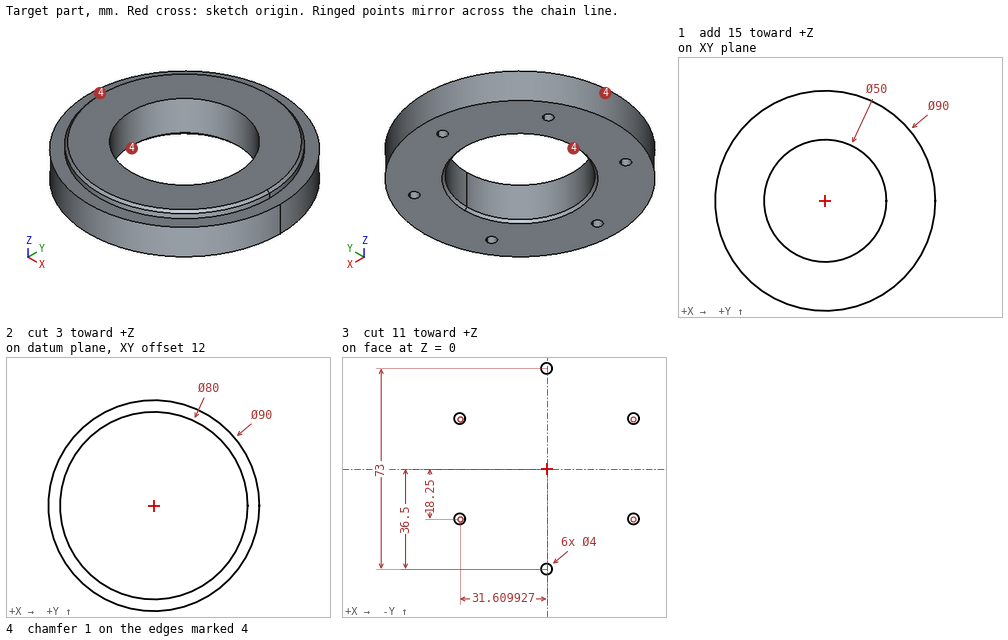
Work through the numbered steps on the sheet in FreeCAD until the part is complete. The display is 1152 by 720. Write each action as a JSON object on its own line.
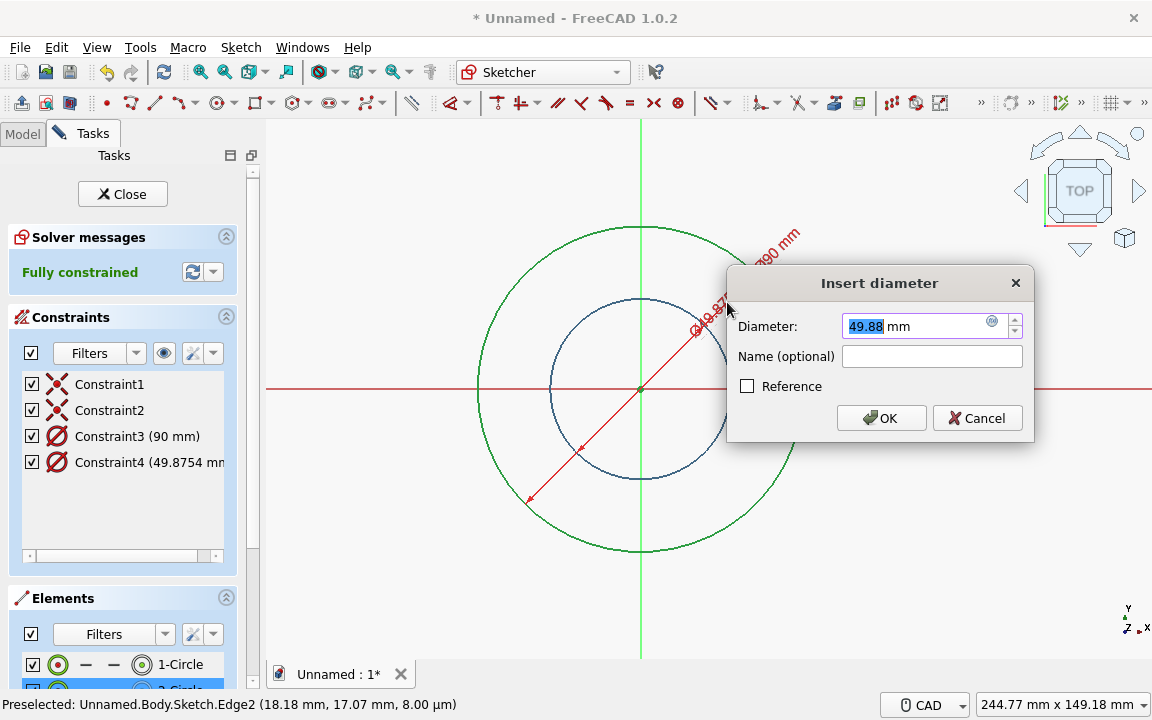
{"action": "type", "text": "50"}
{"action": "key", "text": "Return"}
{"action": "key", "text": "Escape"}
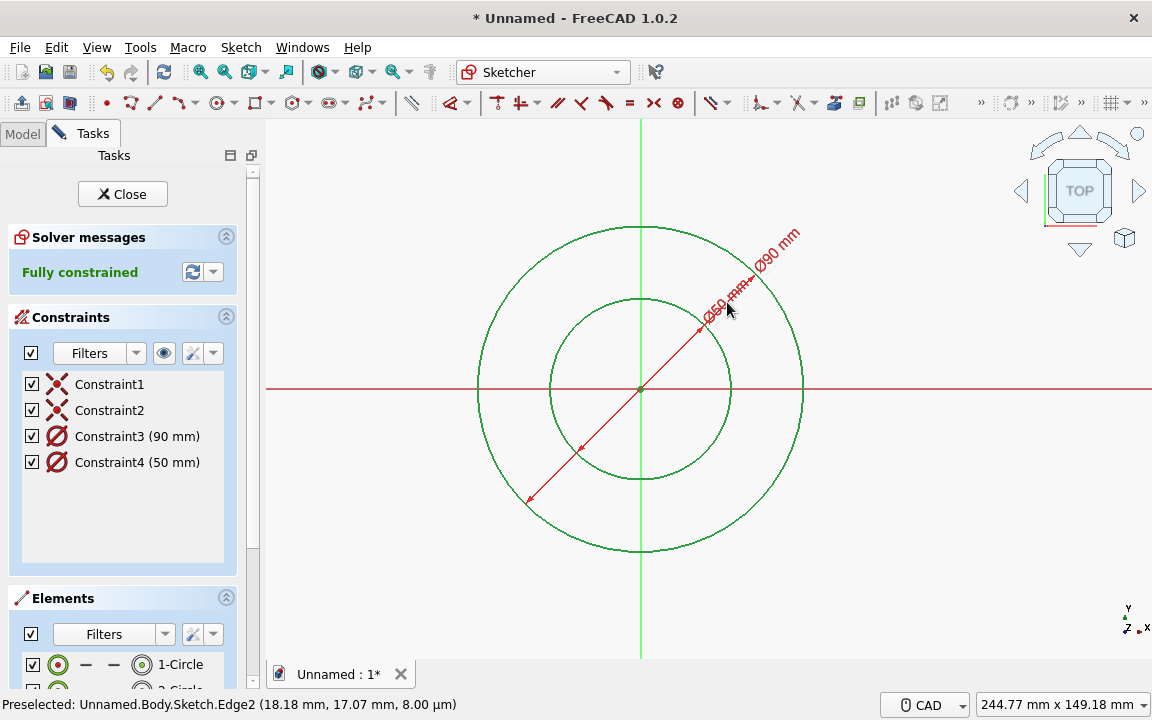
{"action": "left_click", "coordinate": [123, 194]}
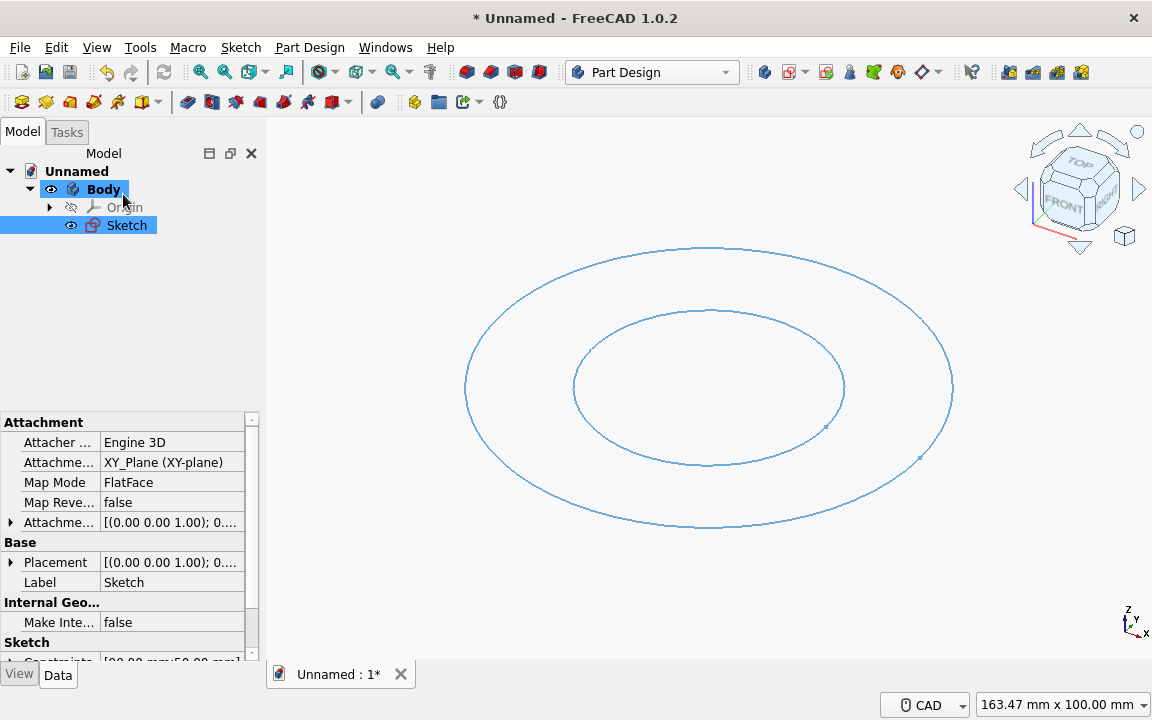
{"action": "left_click", "coordinate": [22, 102]}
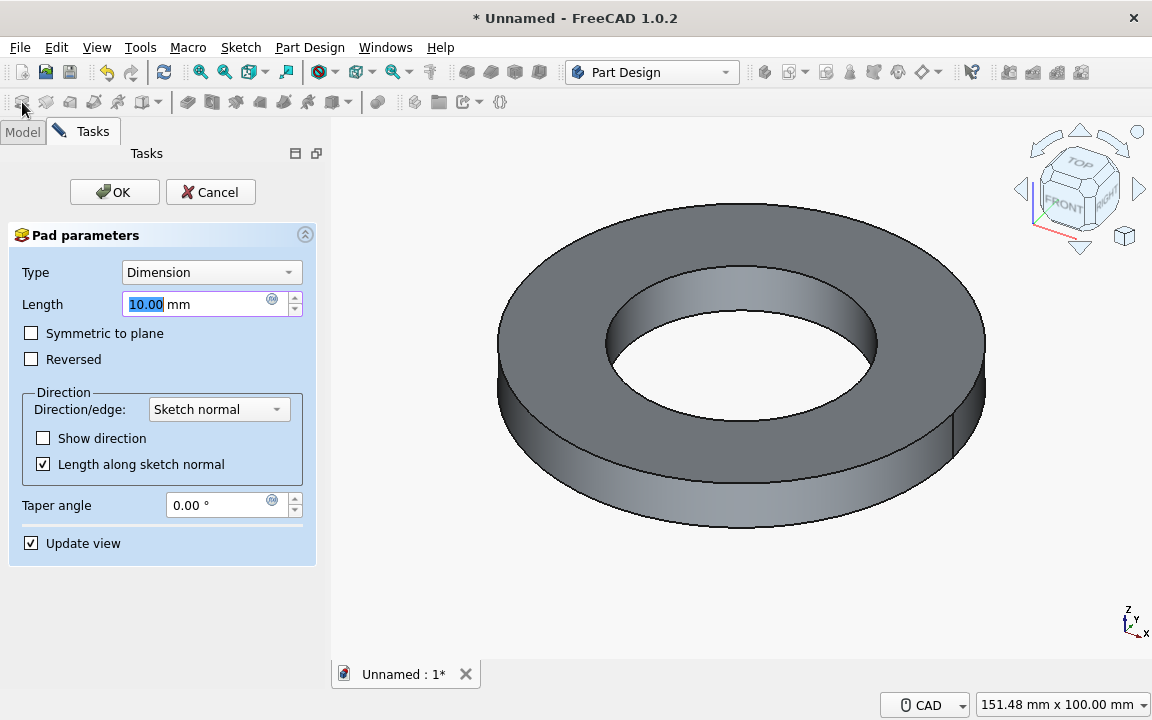
{"action": "type", "text": "15"}
{"action": "key", "text": "Tab"}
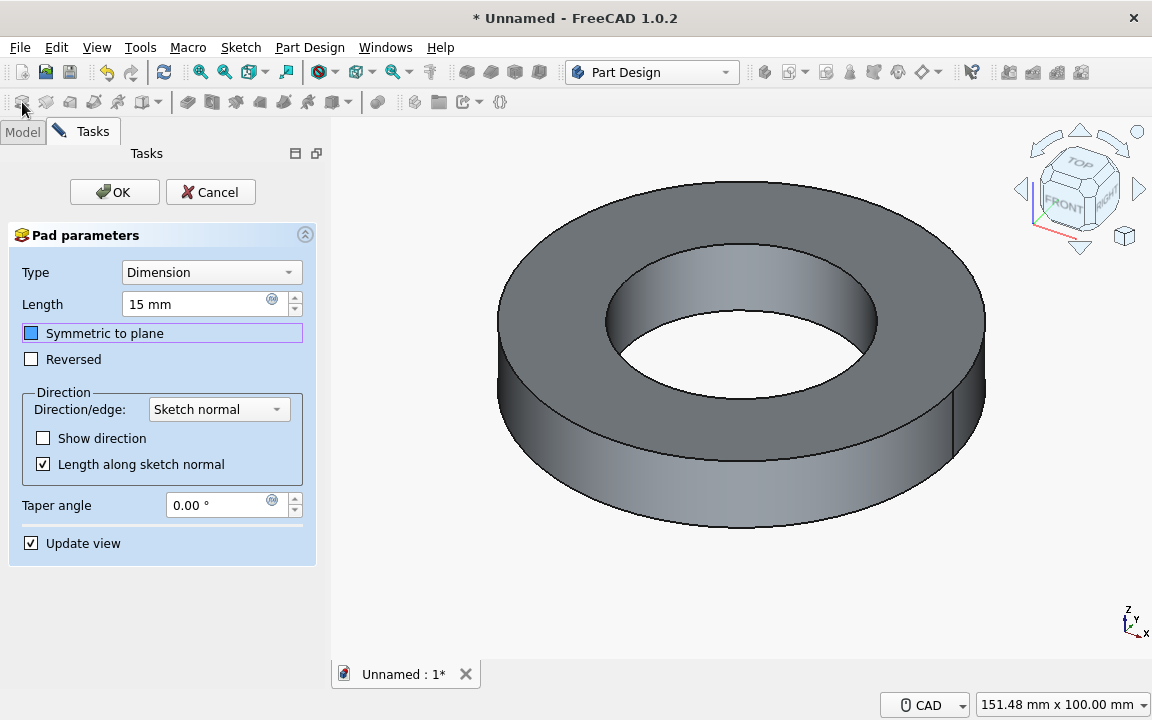
{"action": "left_click", "coordinate": [115, 192]}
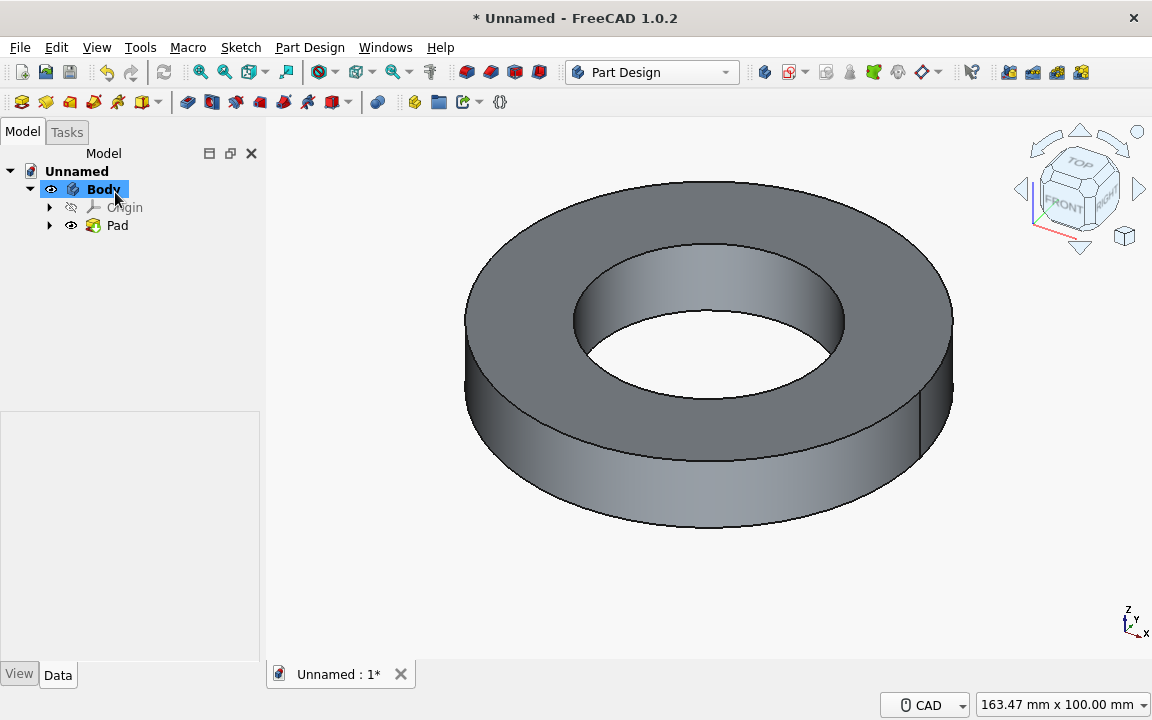
{"action": "left_click", "coordinate": [50, 207]}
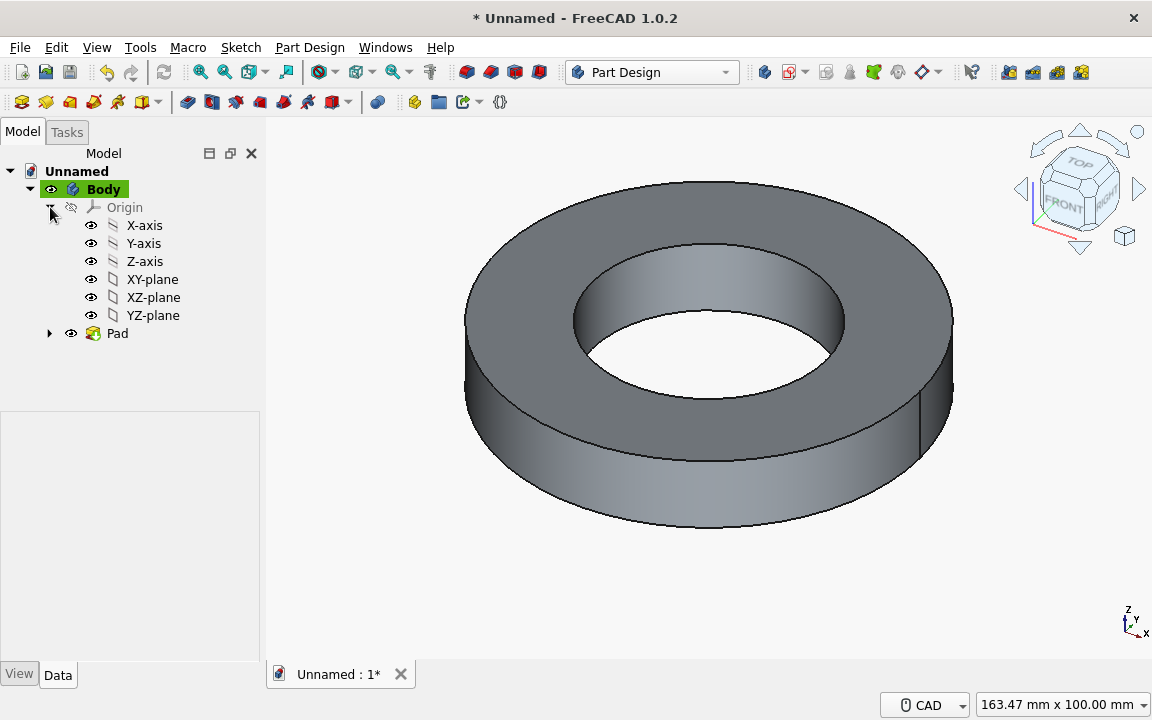
{"action": "left_click", "coordinate": [136, 279]}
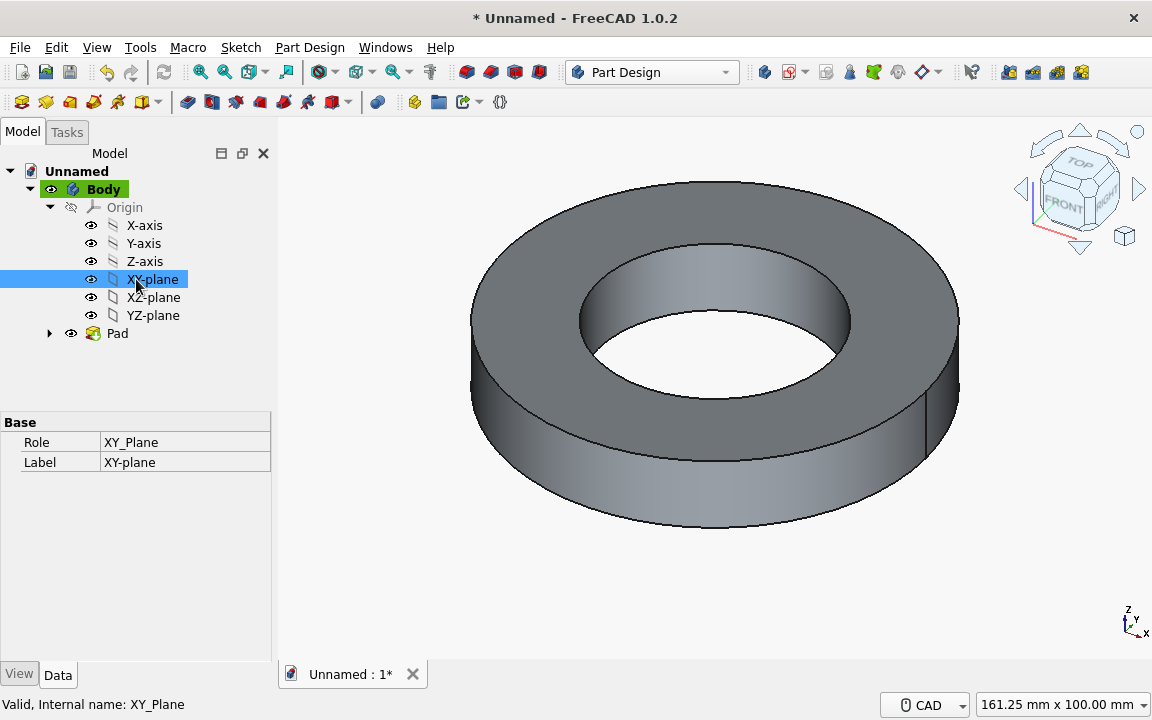
{"action": "left_click", "coordinate": [922, 72]}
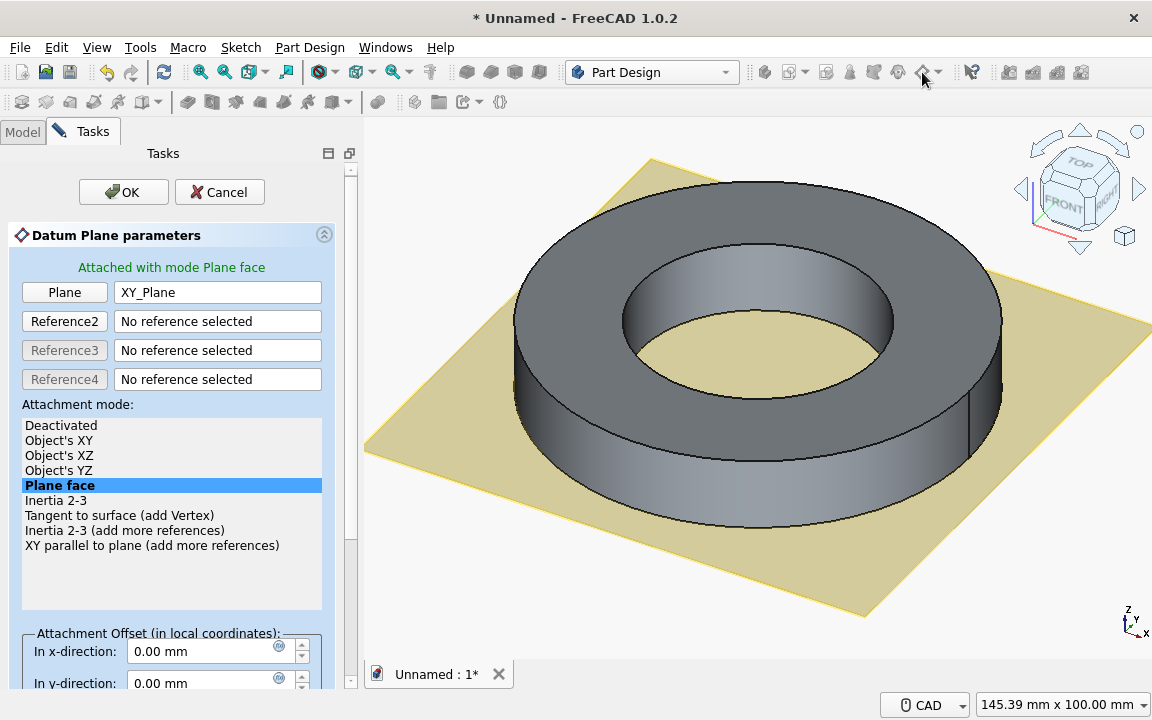
{"action": "scroll", "coordinate": [351, 426], "scroll_direction": "down", "scroll_amount": 2}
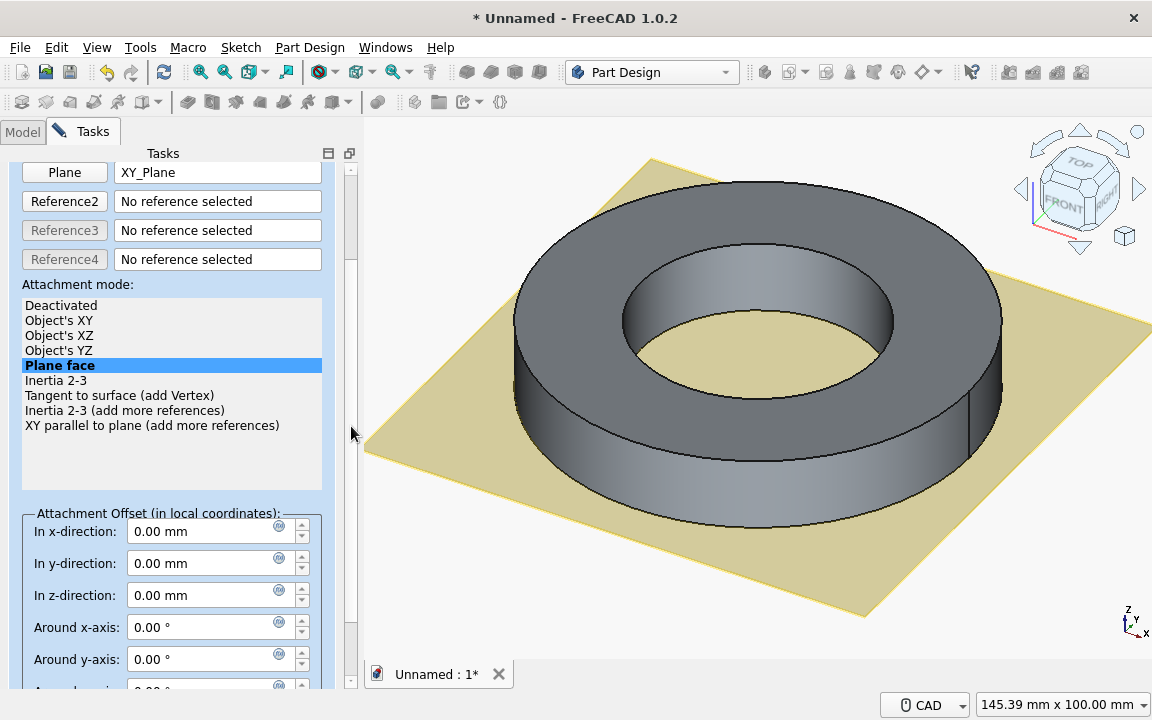
{"action": "triple_click", "coordinate": [210, 595]}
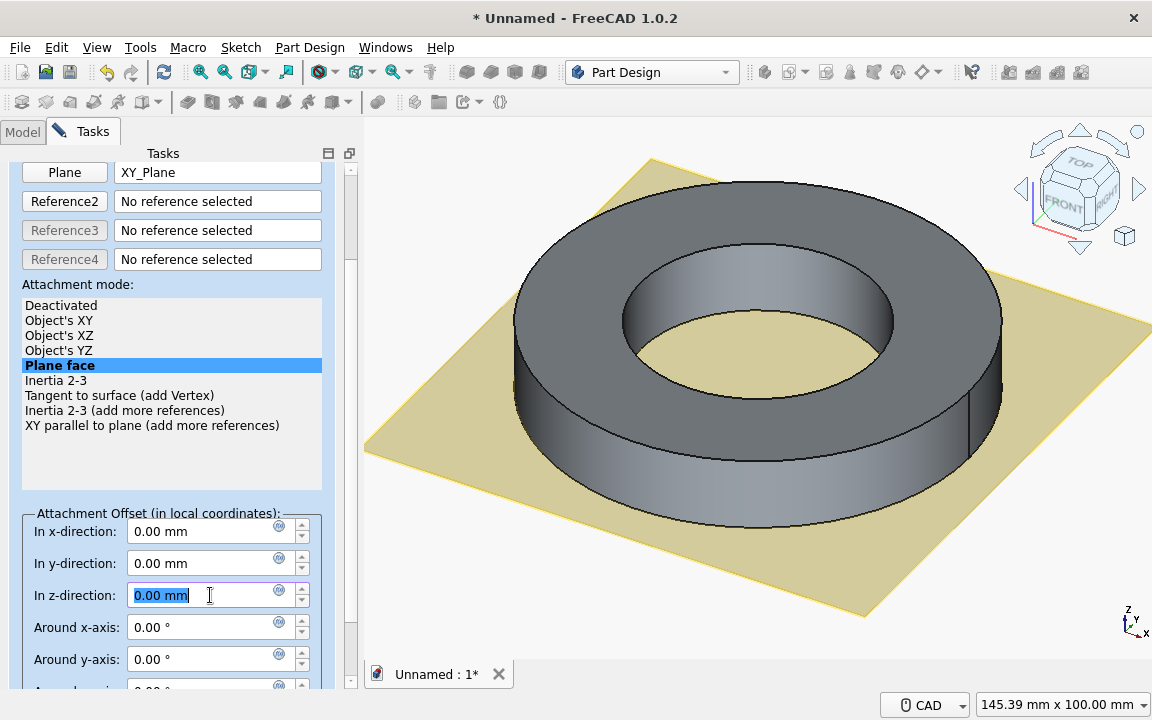
{"action": "type", "text": "12"}
{"action": "key", "text": "Tab"}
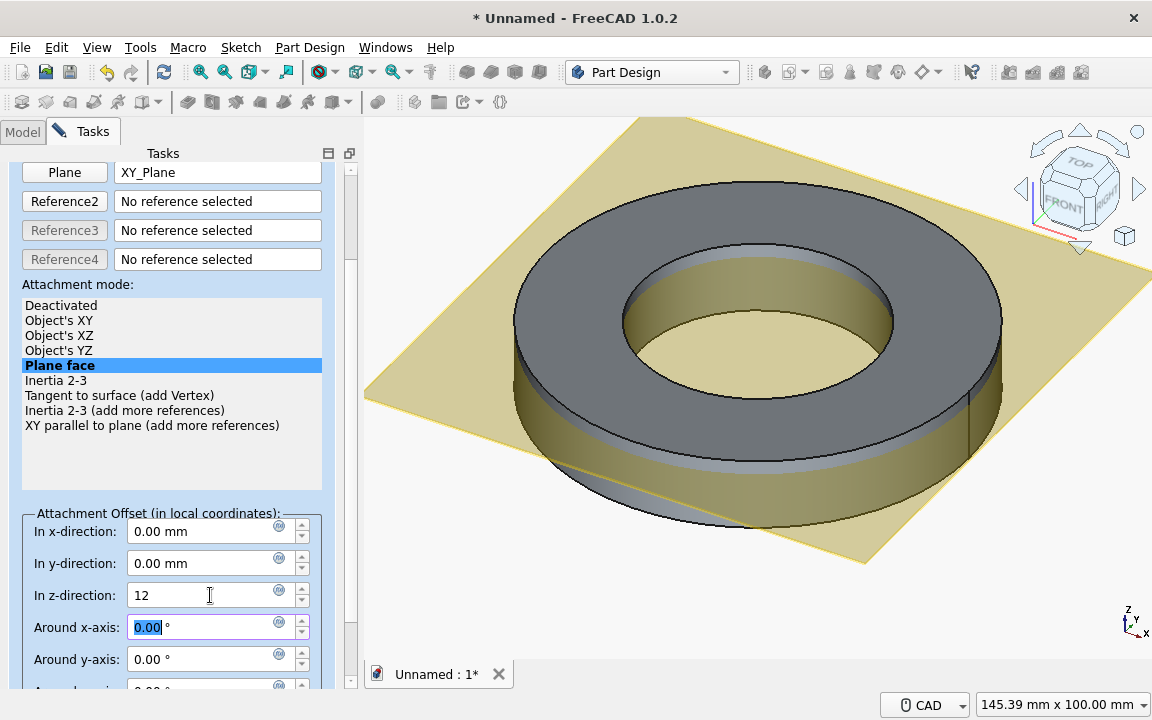
{"action": "scroll", "coordinate": [351, 426], "scroll_direction": "up", "scroll_amount": 3}